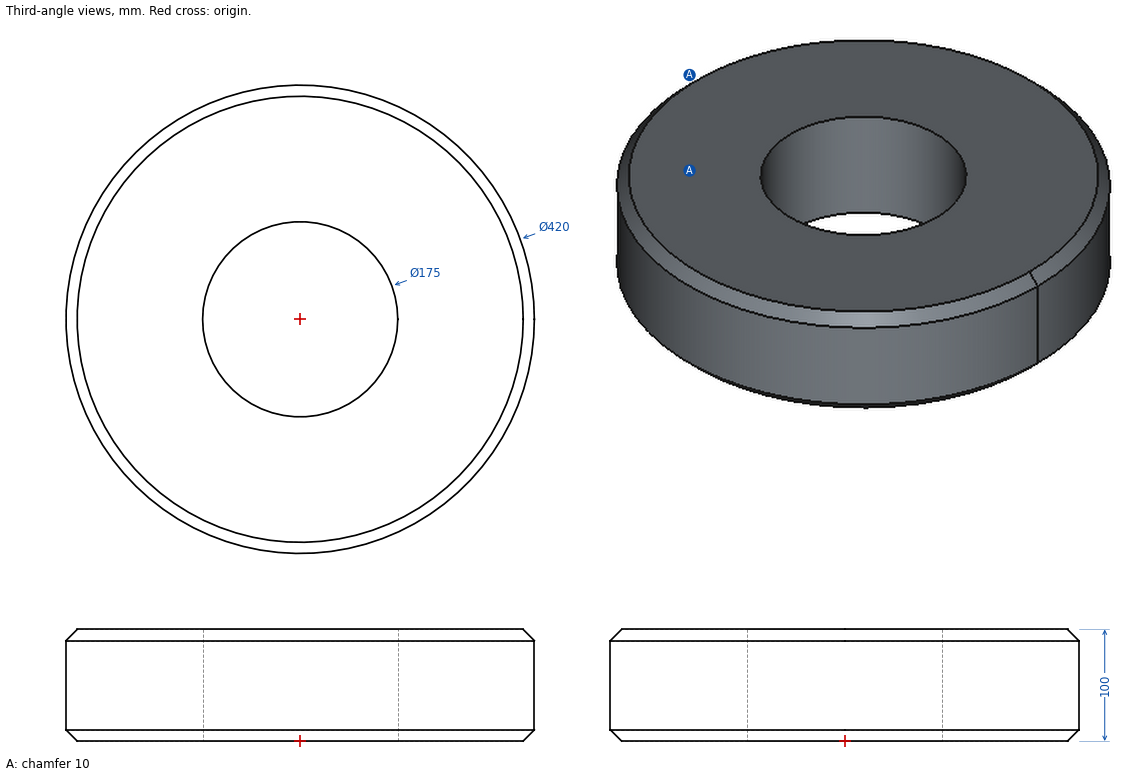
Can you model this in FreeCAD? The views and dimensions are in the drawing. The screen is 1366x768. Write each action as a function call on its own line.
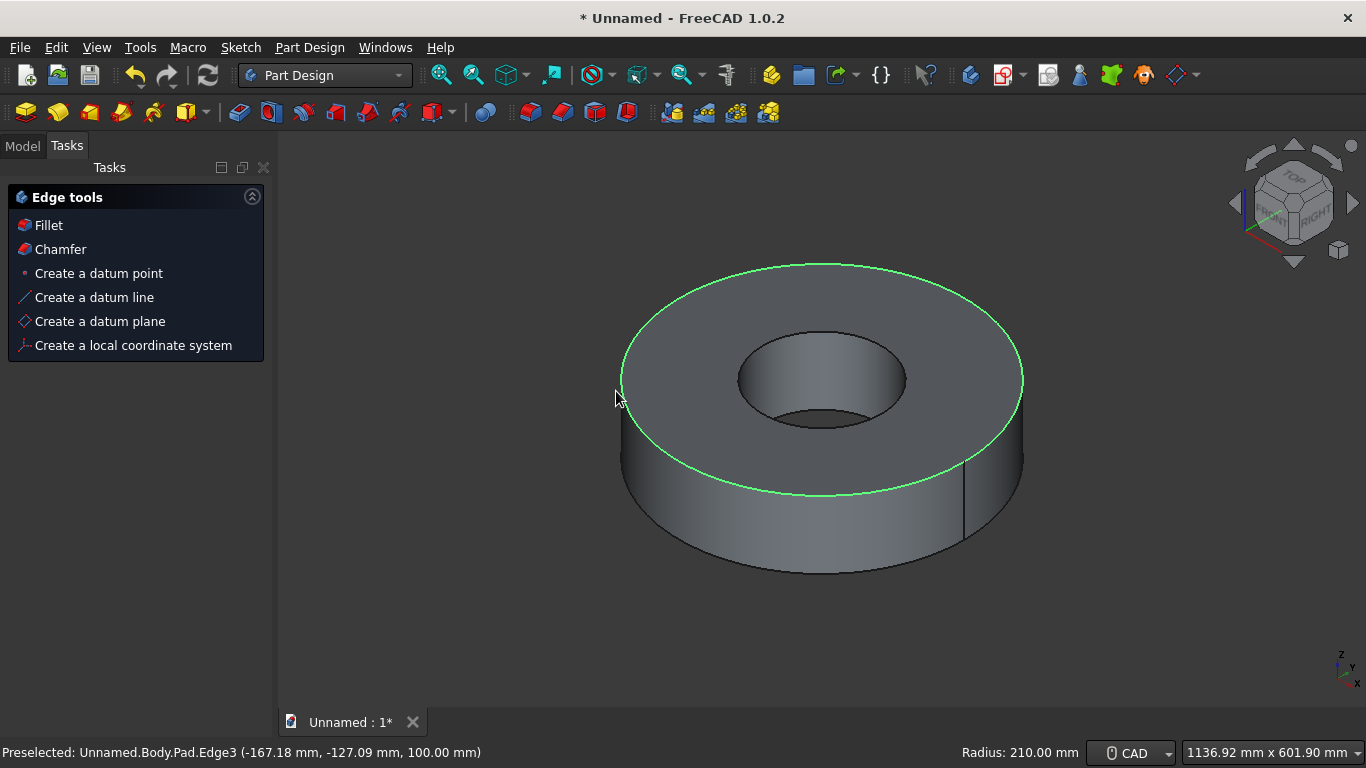
key(2)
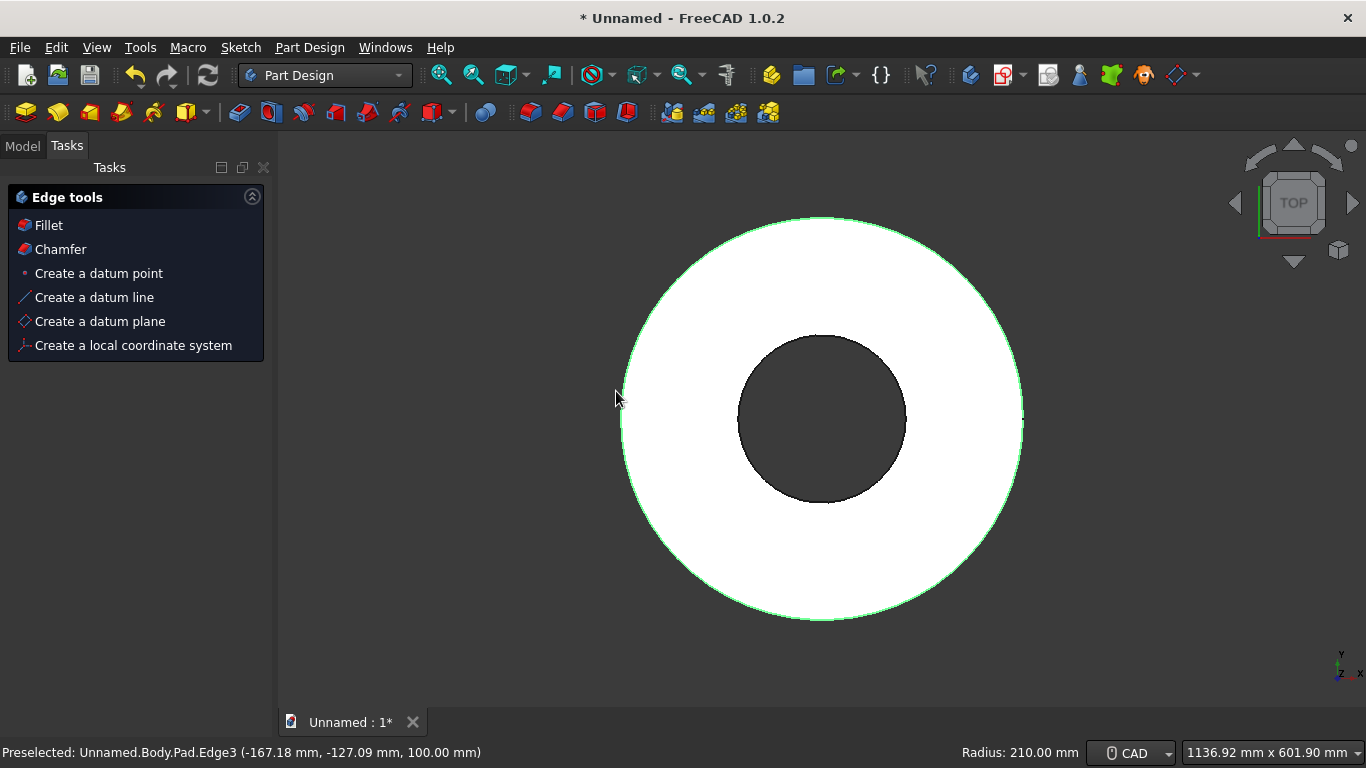
key(1)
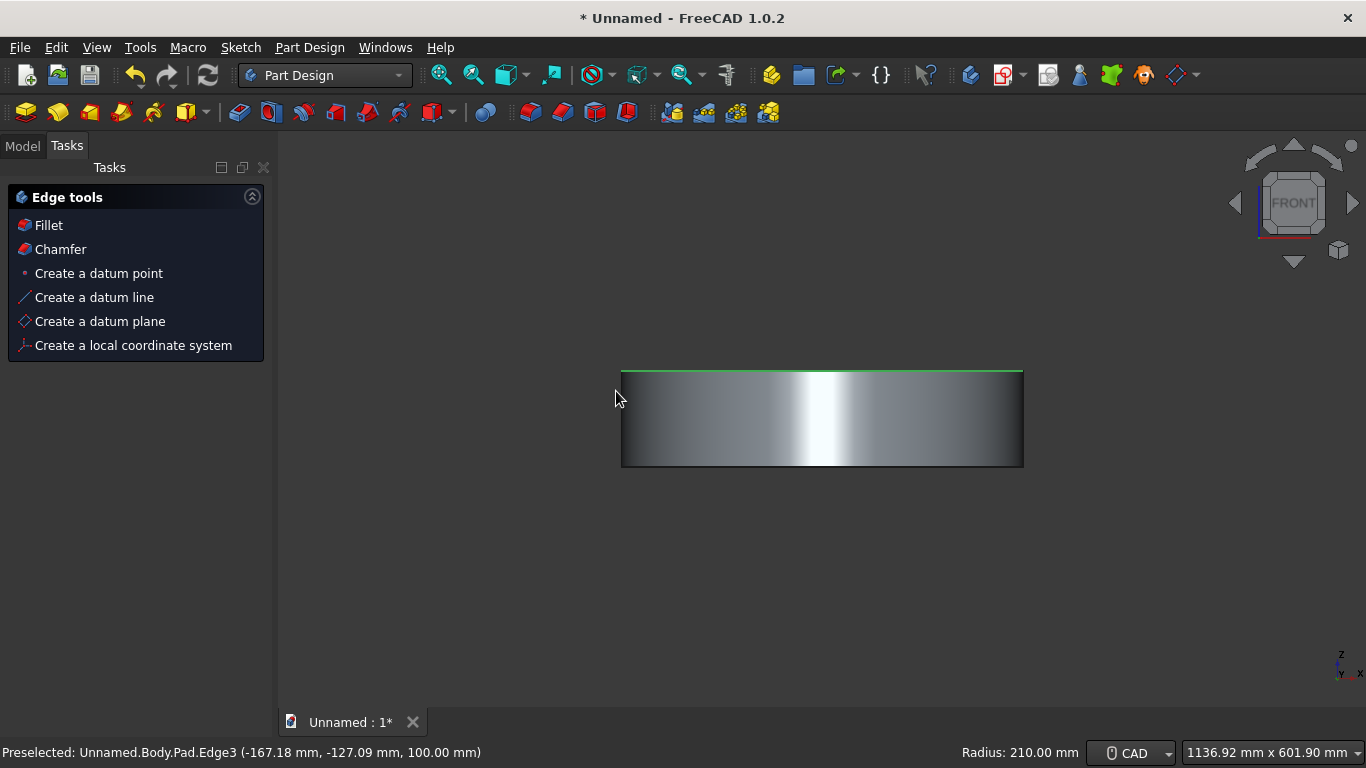
key(v)
key(f)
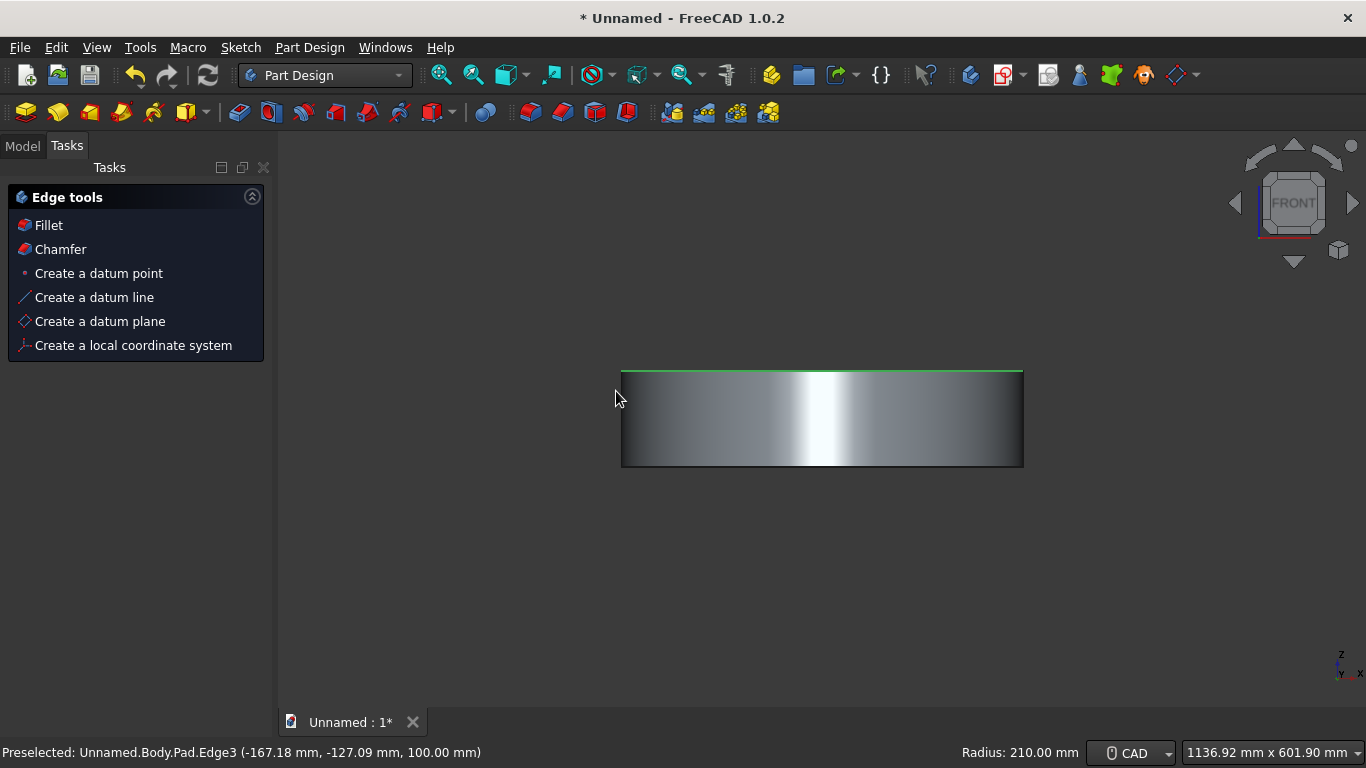
click(659, 466, ctrl)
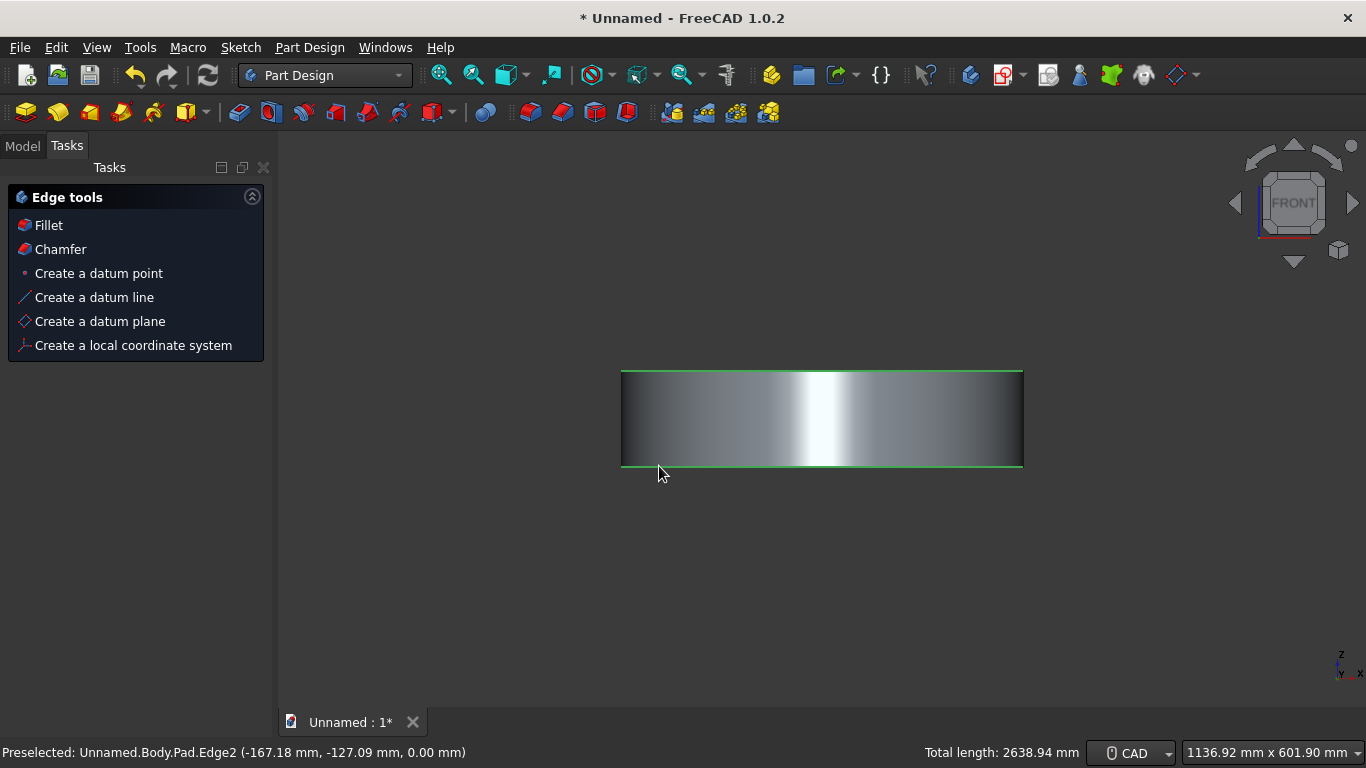
click(564, 112)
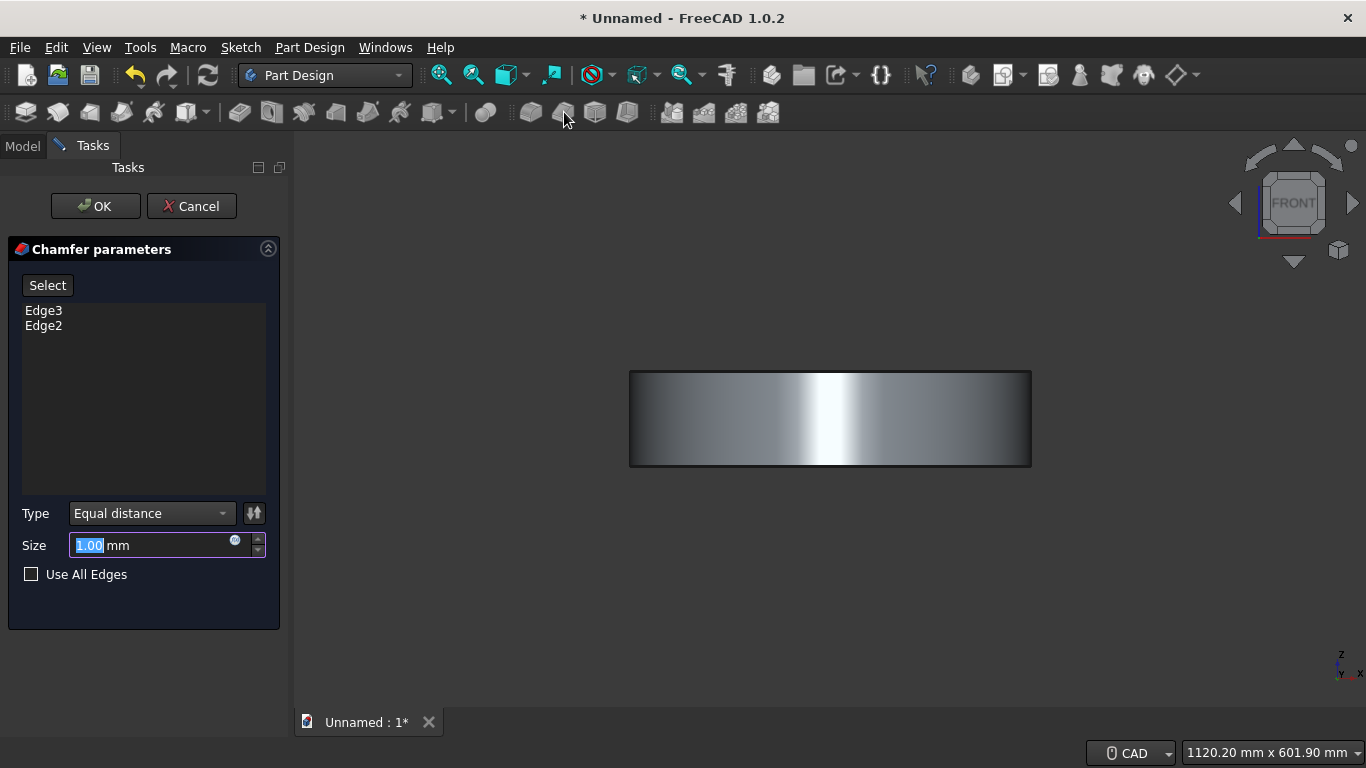
text(10)
key(Tab)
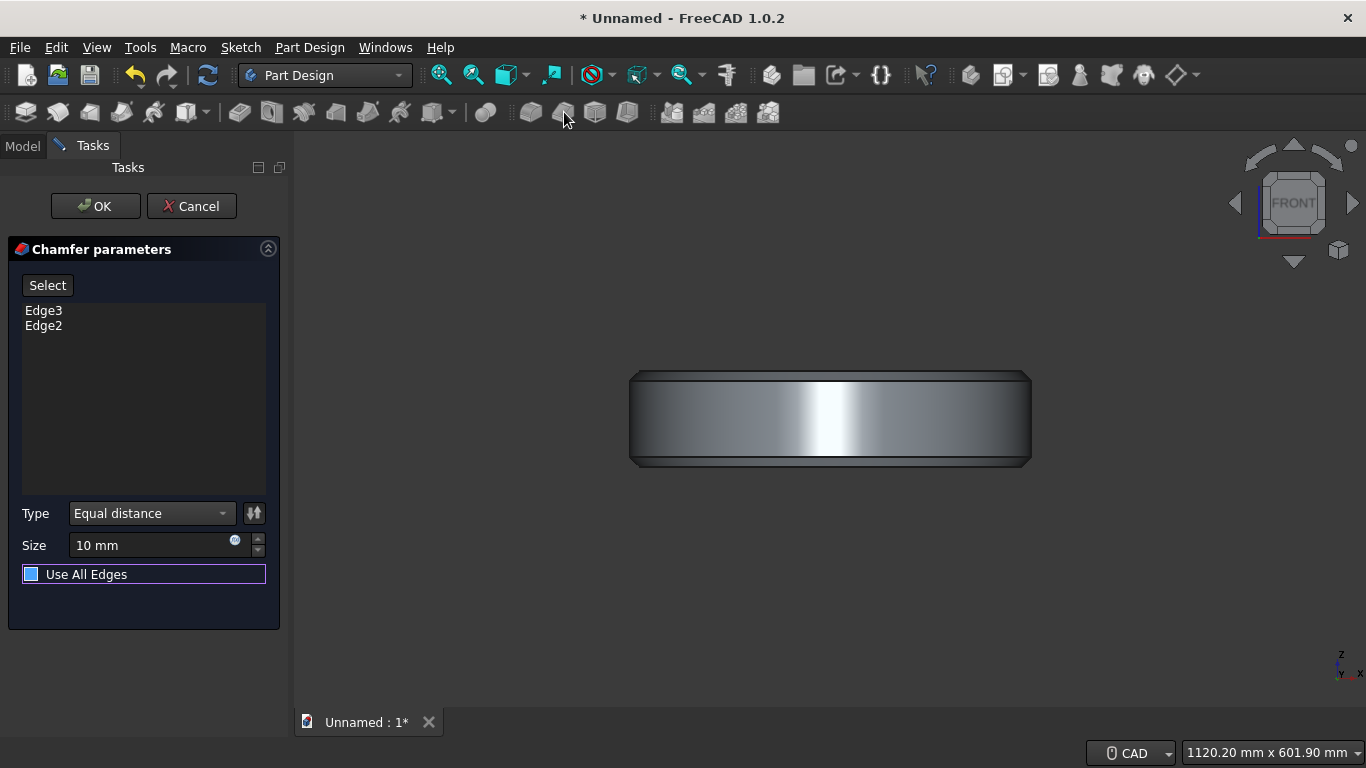
click(96, 206)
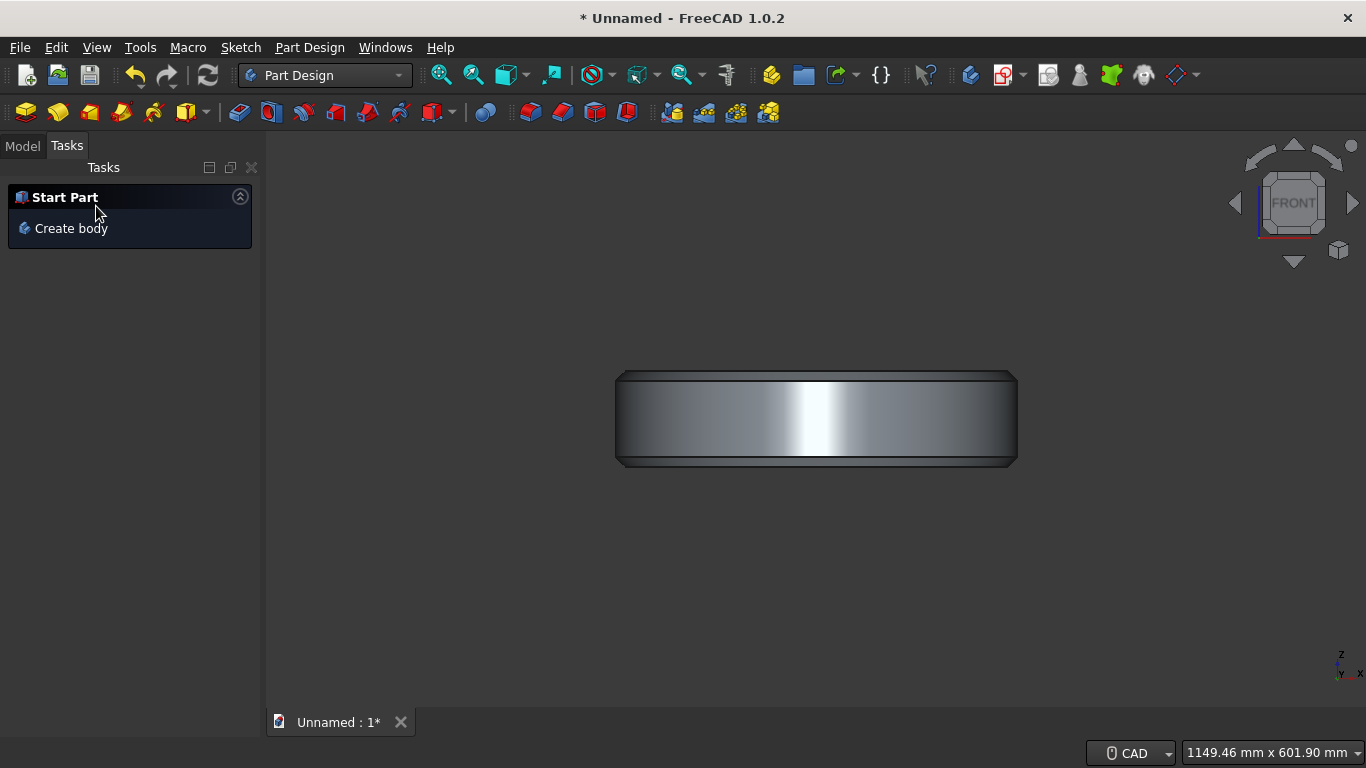
key(0)